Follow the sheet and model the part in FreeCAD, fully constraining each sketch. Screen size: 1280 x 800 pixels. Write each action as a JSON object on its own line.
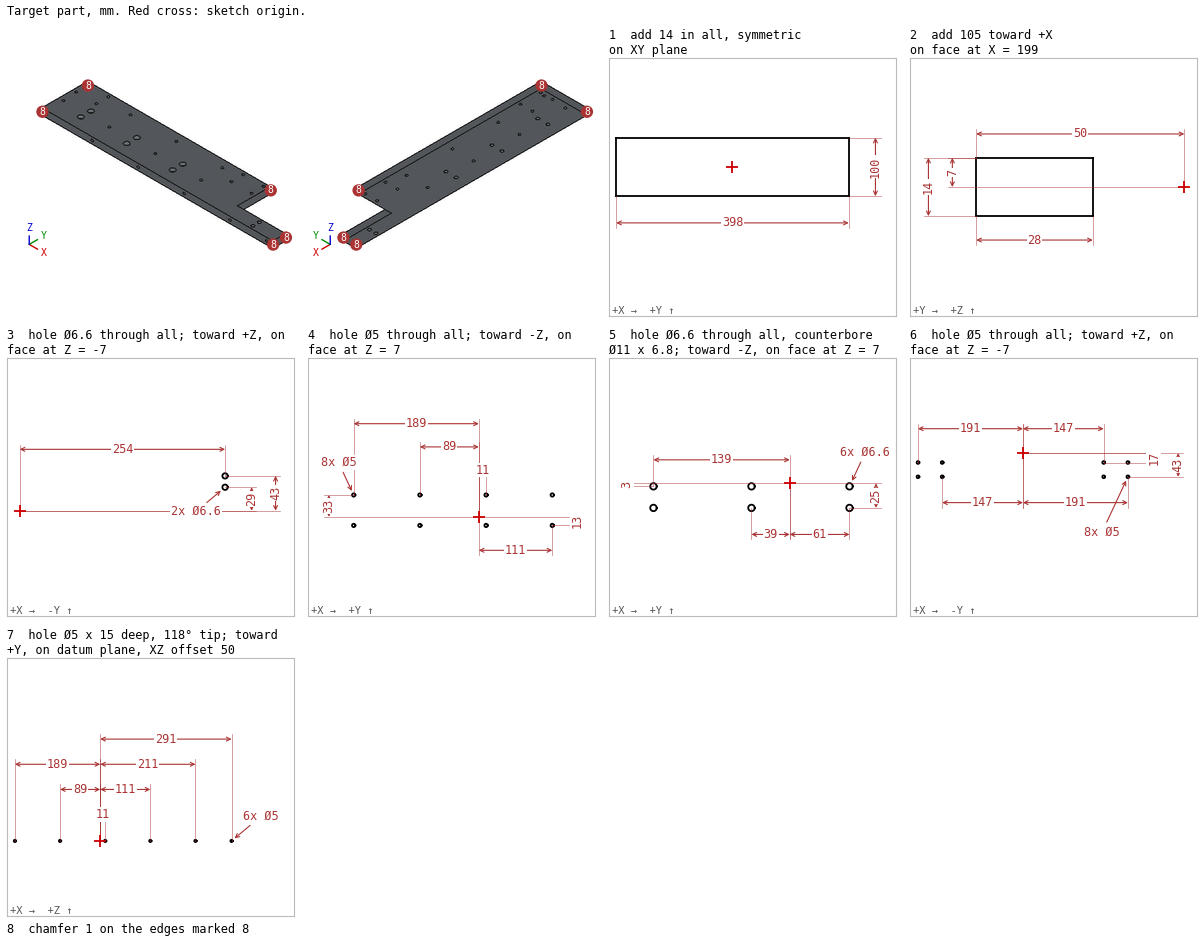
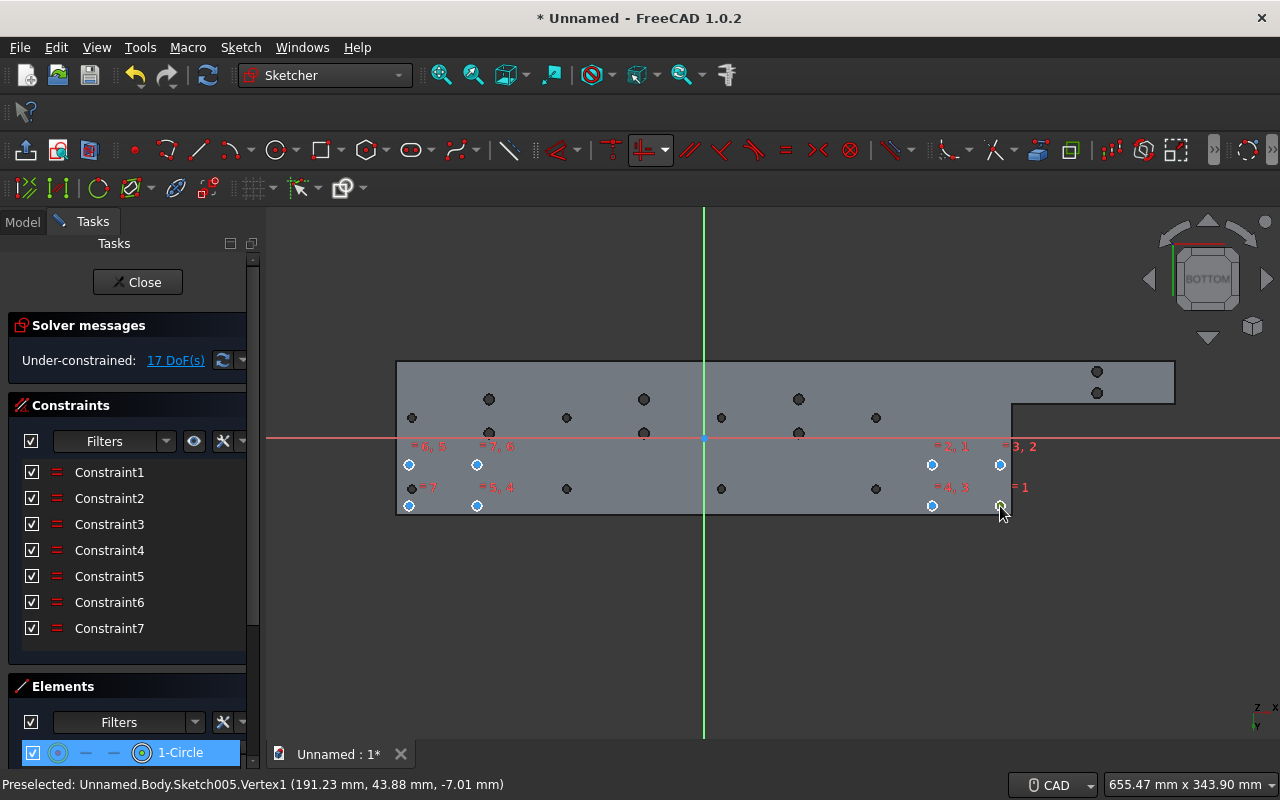
{"action": "left_click", "coordinate": [1000, 465]}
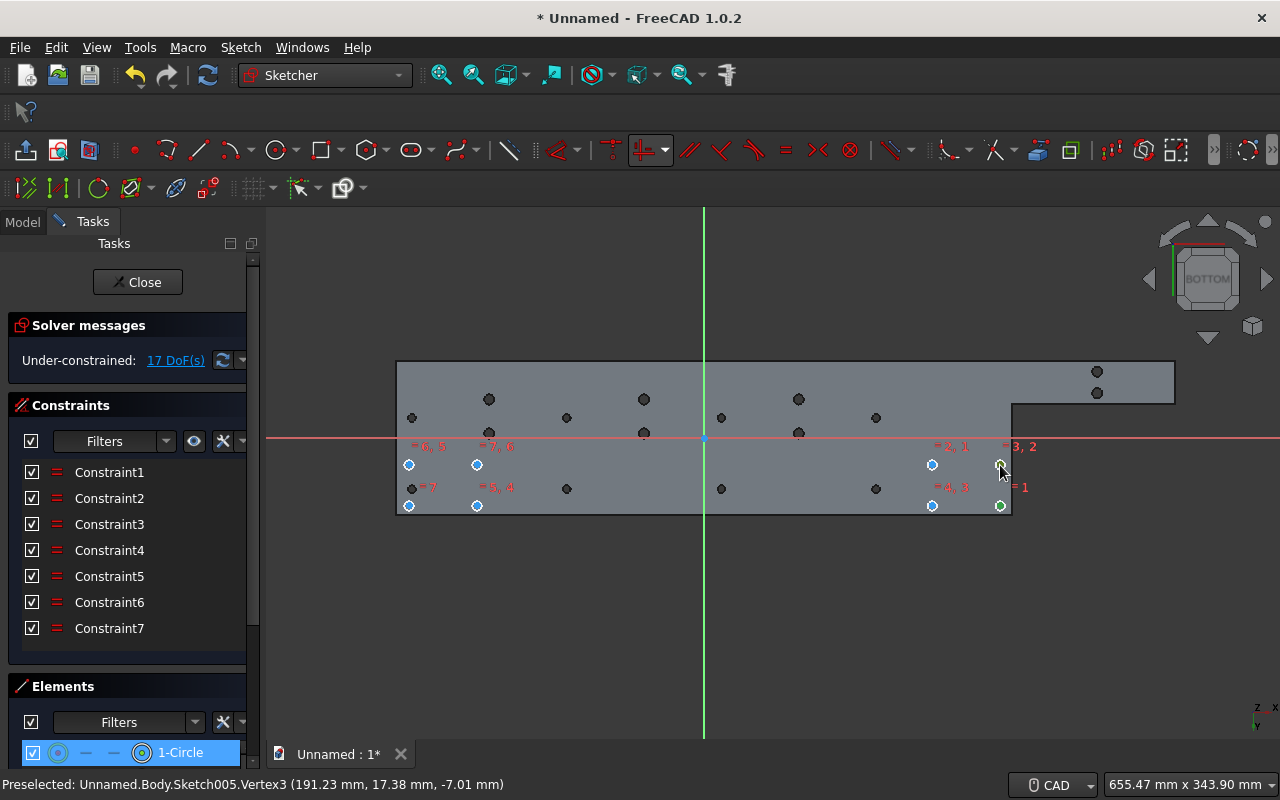
{"action": "left_click", "coordinate": [668, 150]}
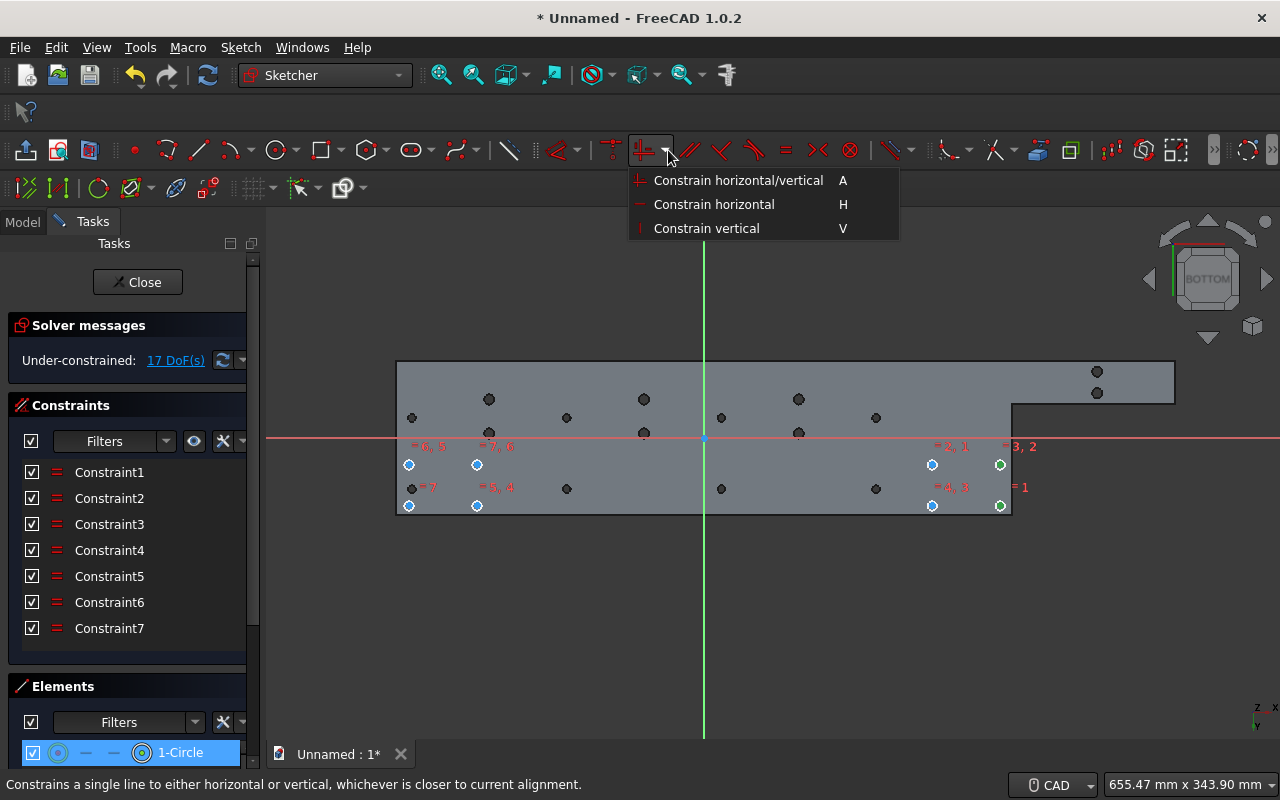
{"action": "left_click", "coordinate": [764, 228]}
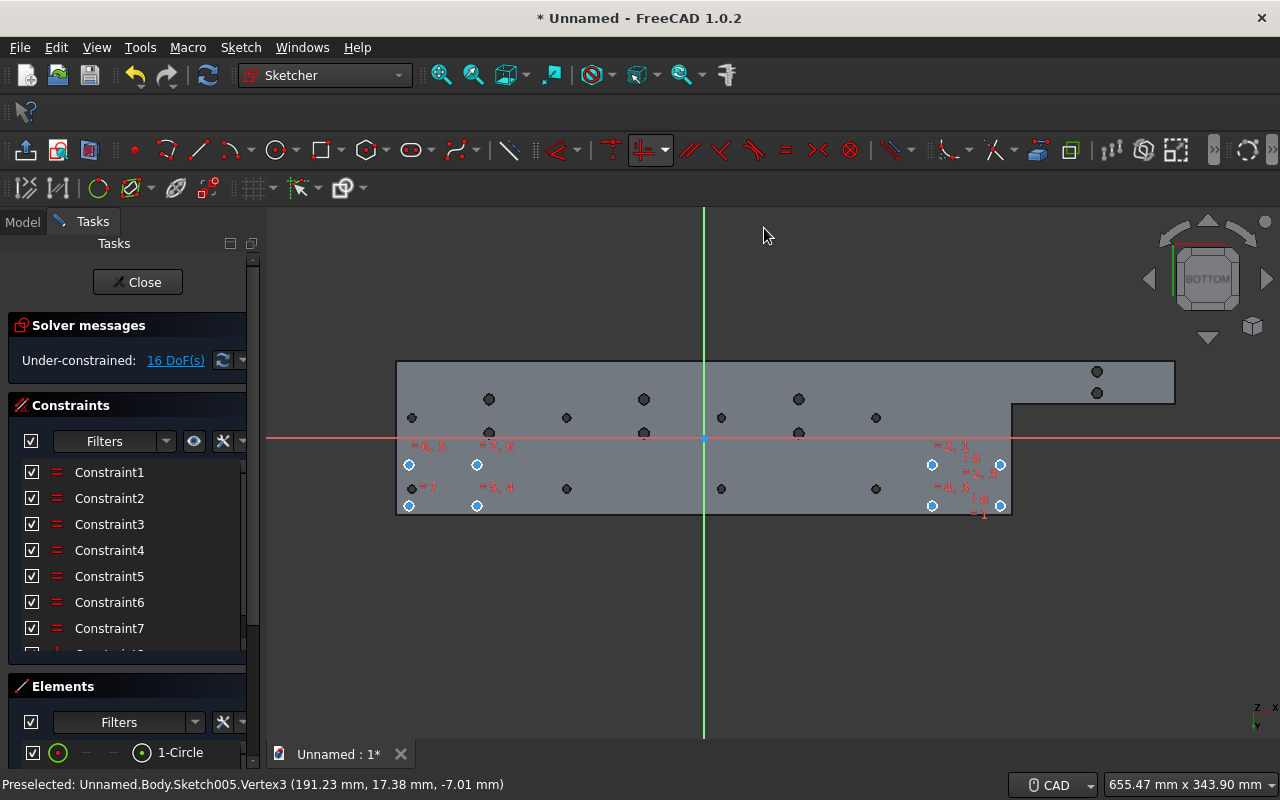
{"action": "left_click", "coordinate": [932, 465]}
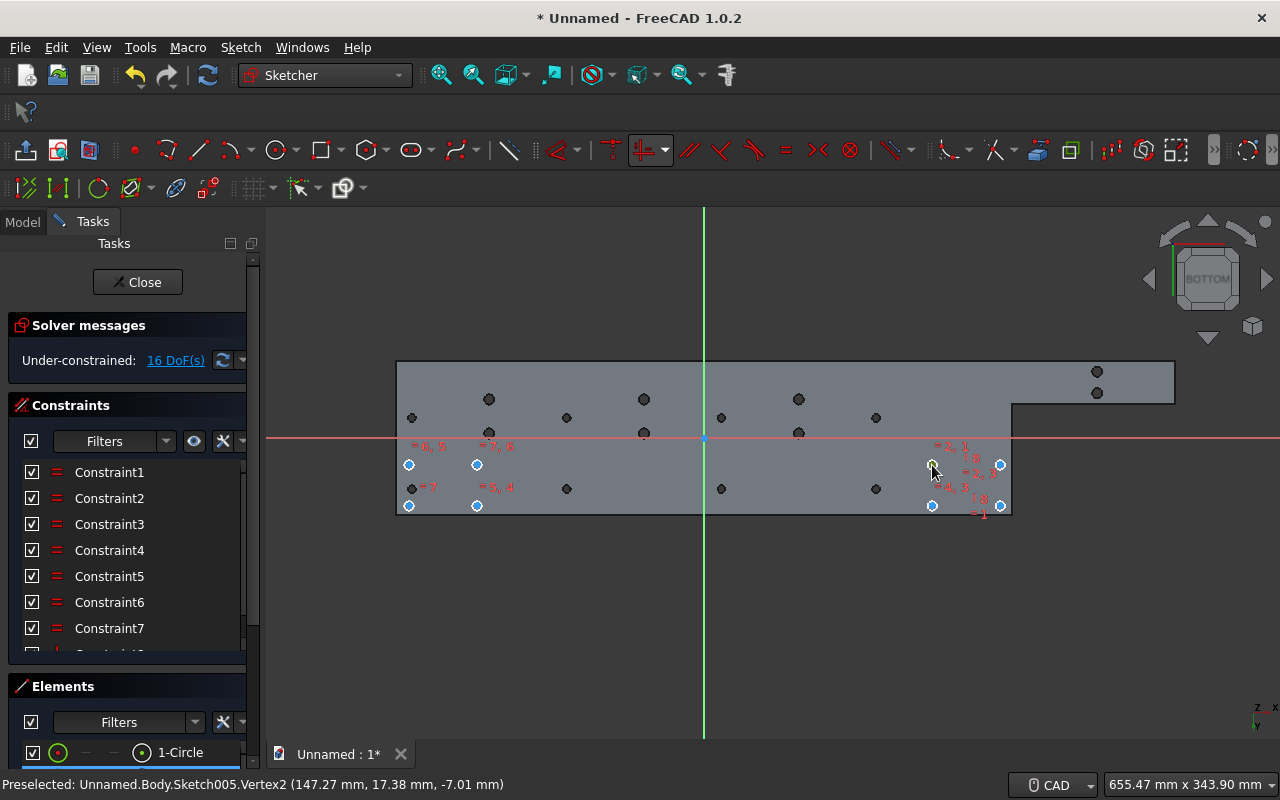
{"action": "left_click", "coordinate": [1000, 465]}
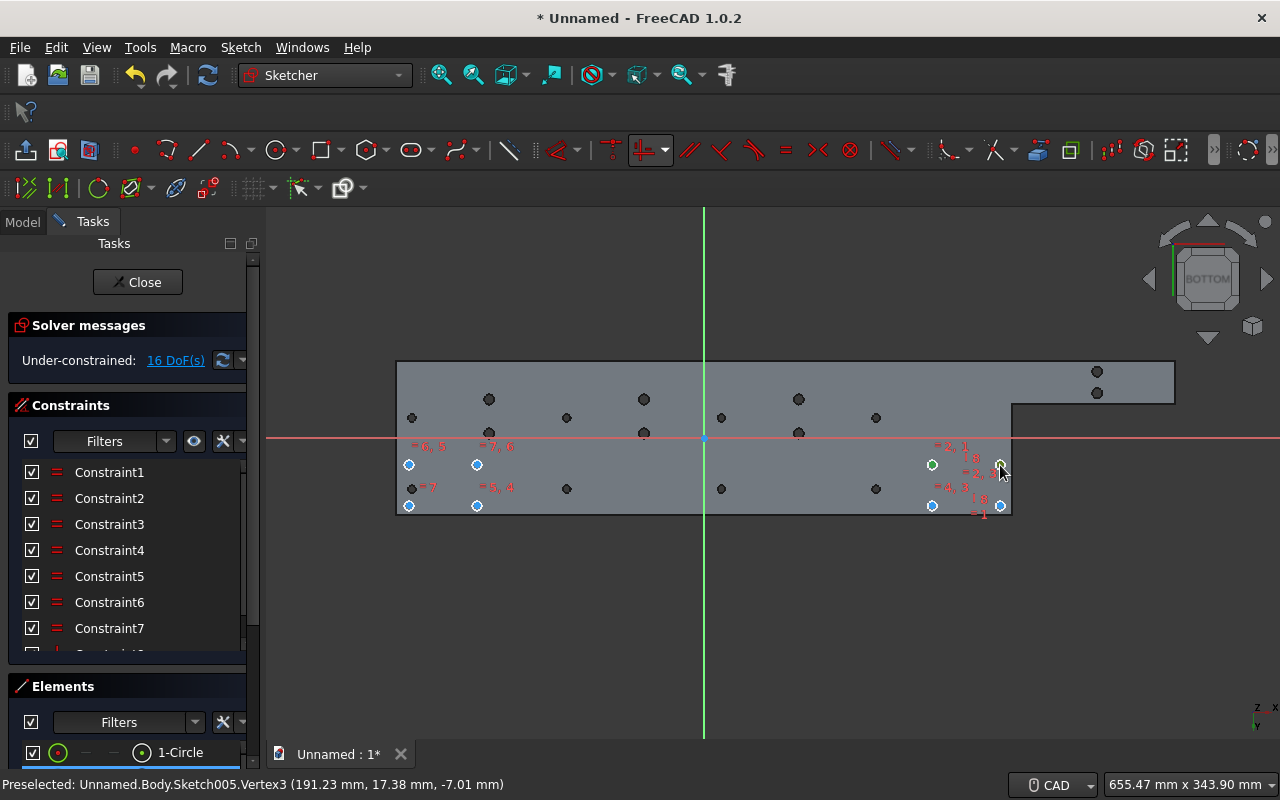
{"action": "key", "text": "h"}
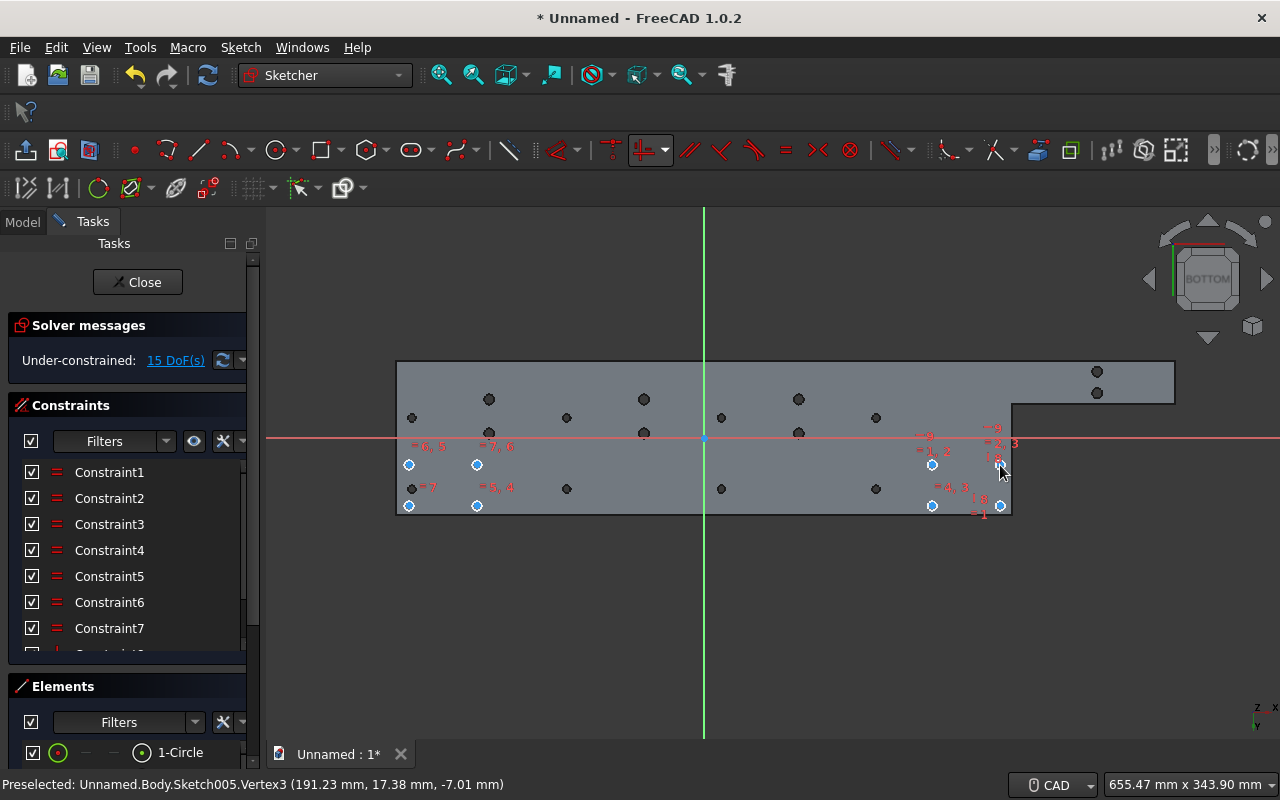
{"action": "left_click", "coordinate": [932, 465]}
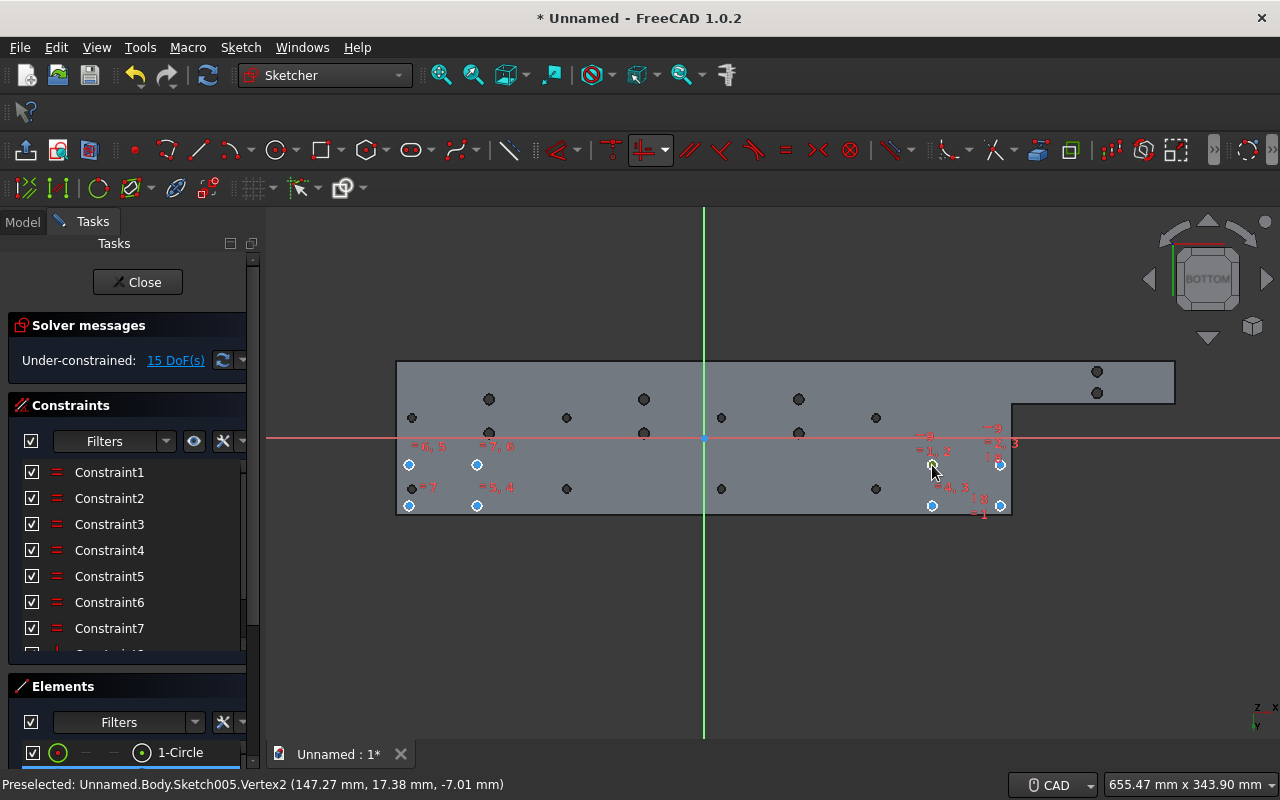
{"action": "left_click", "coordinate": [932, 506]}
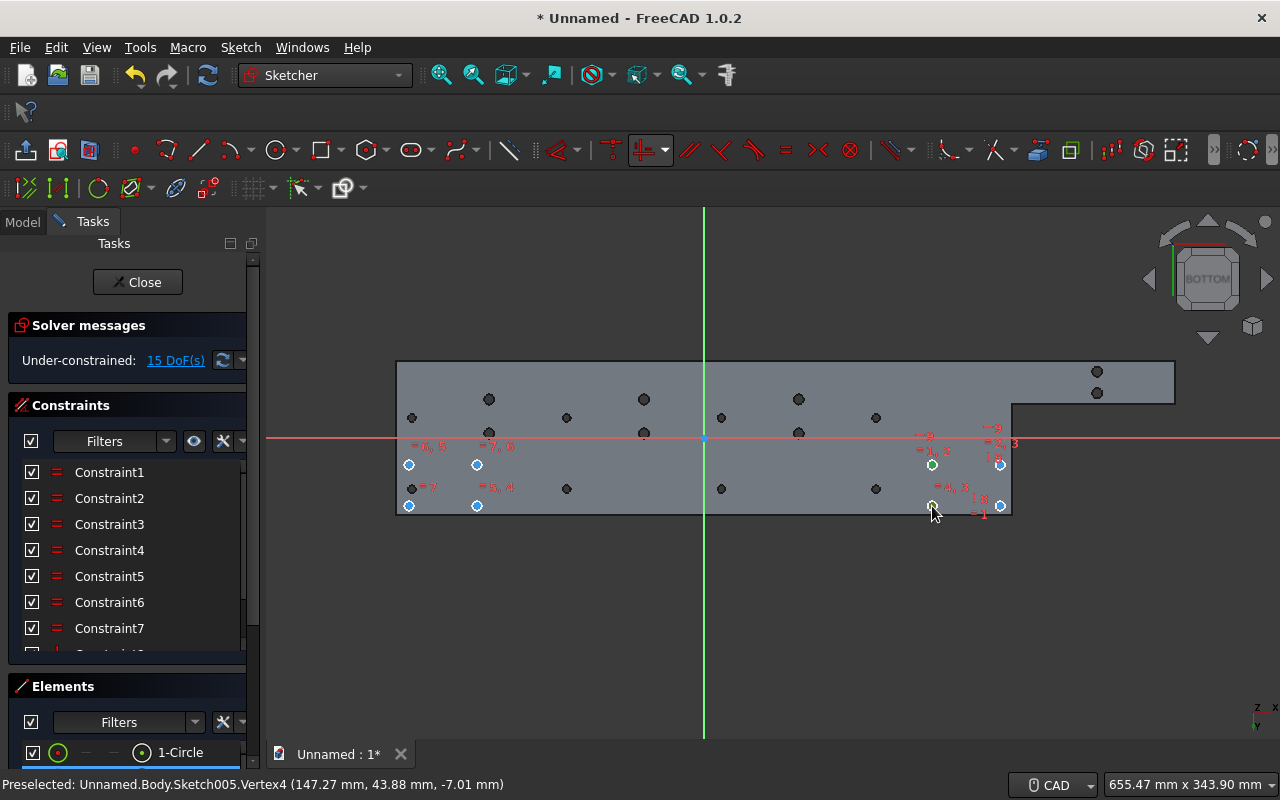
{"action": "key", "text": "v"}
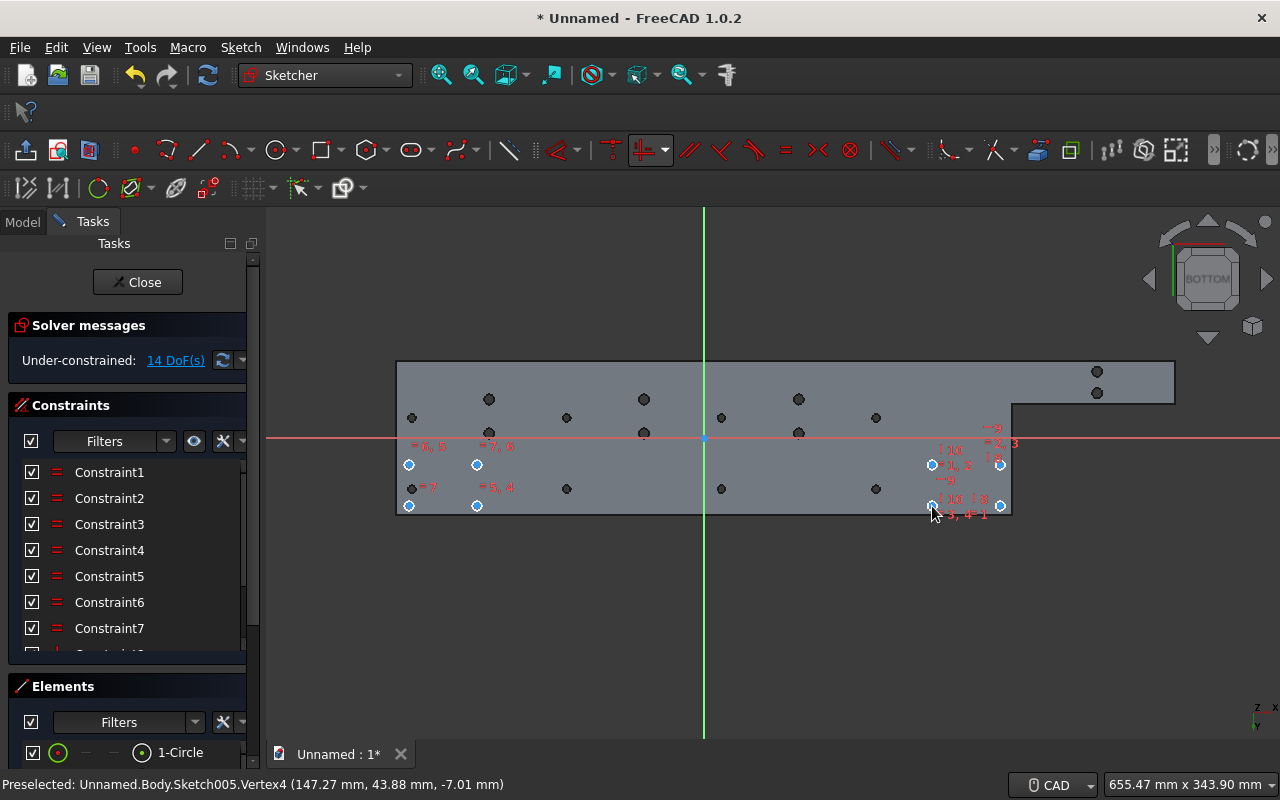
{"action": "left_click", "coordinate": [1000, 506]}